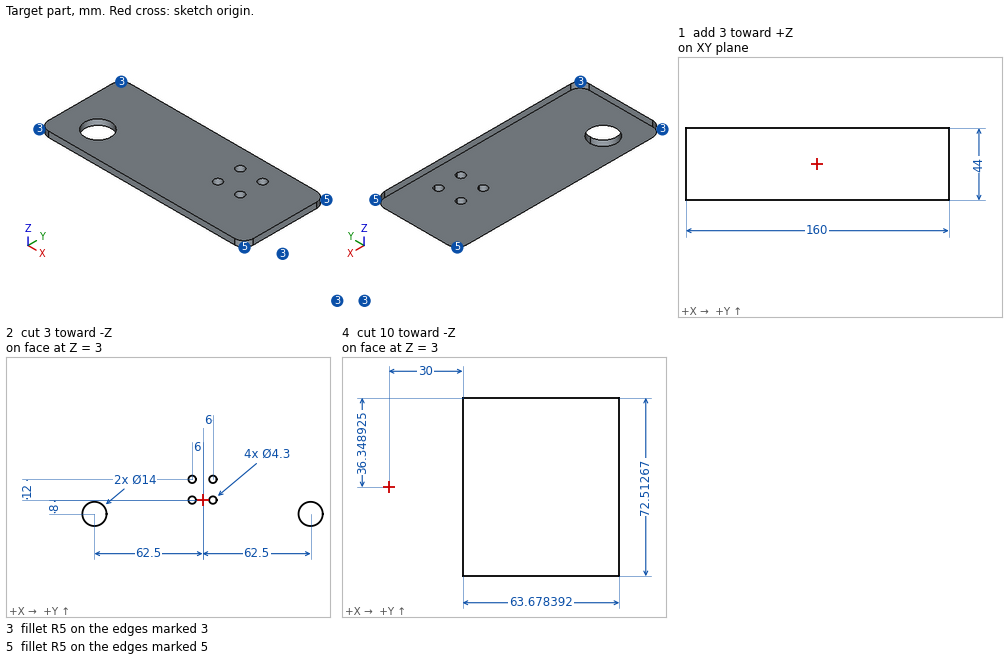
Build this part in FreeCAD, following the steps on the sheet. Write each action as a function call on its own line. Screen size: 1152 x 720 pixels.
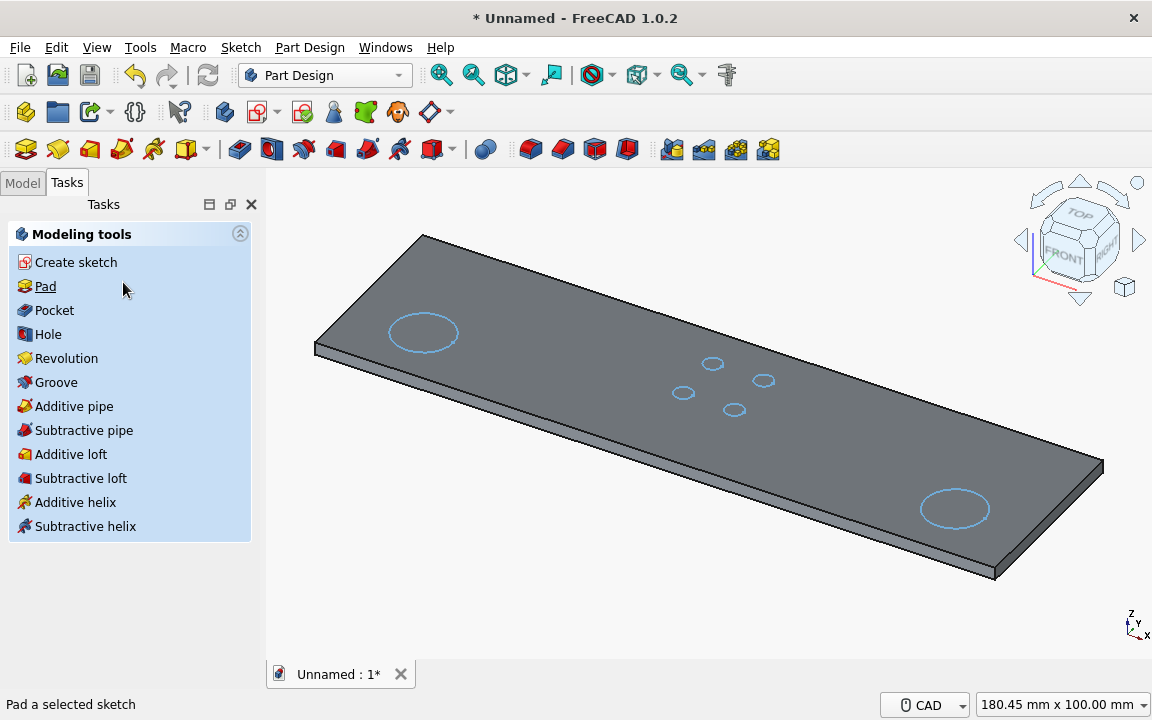
click(240, 150)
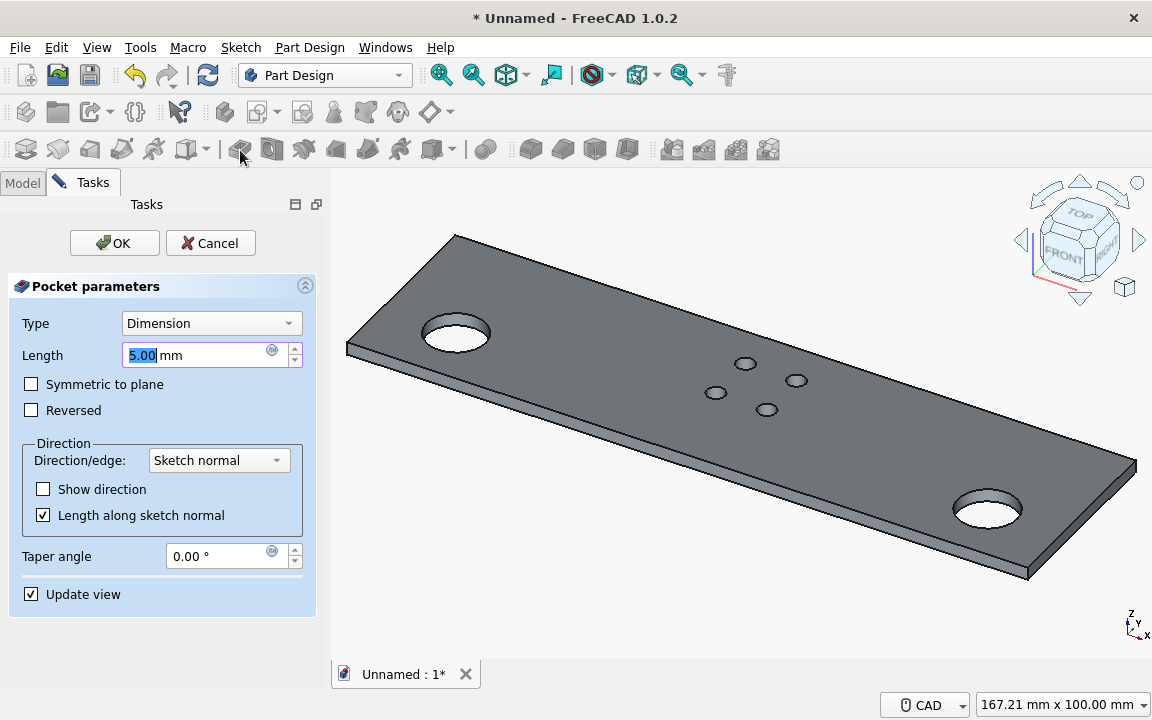
text(3)
key(Tab)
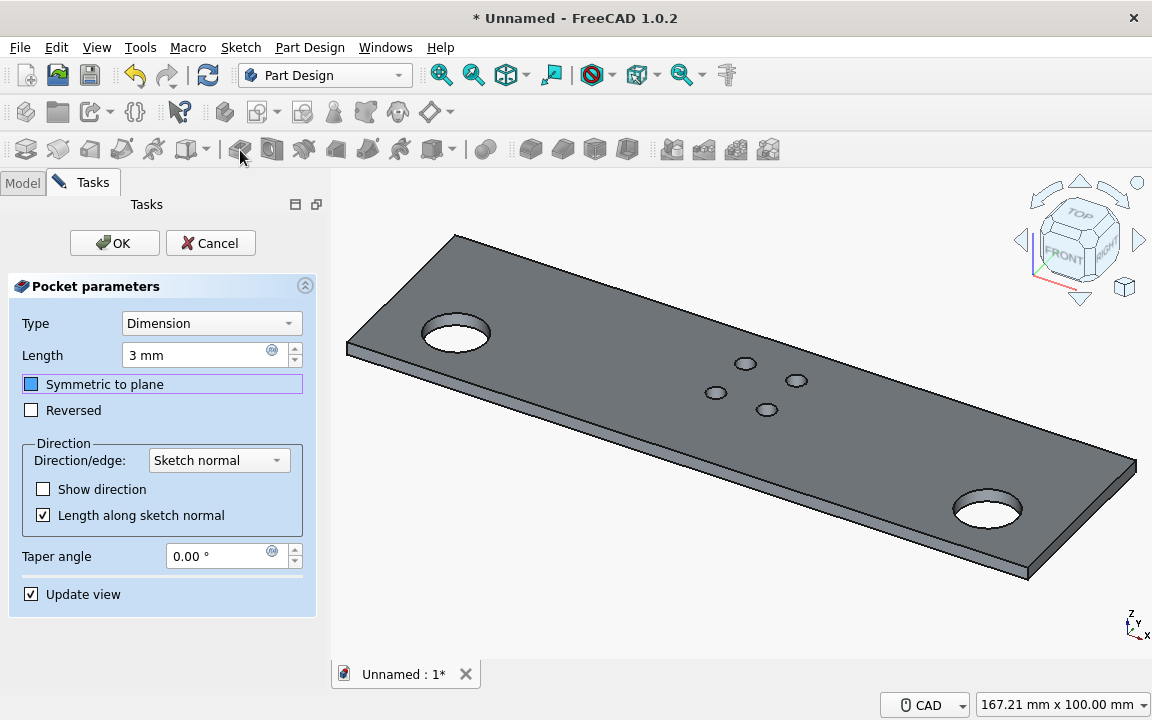
click(115, 243)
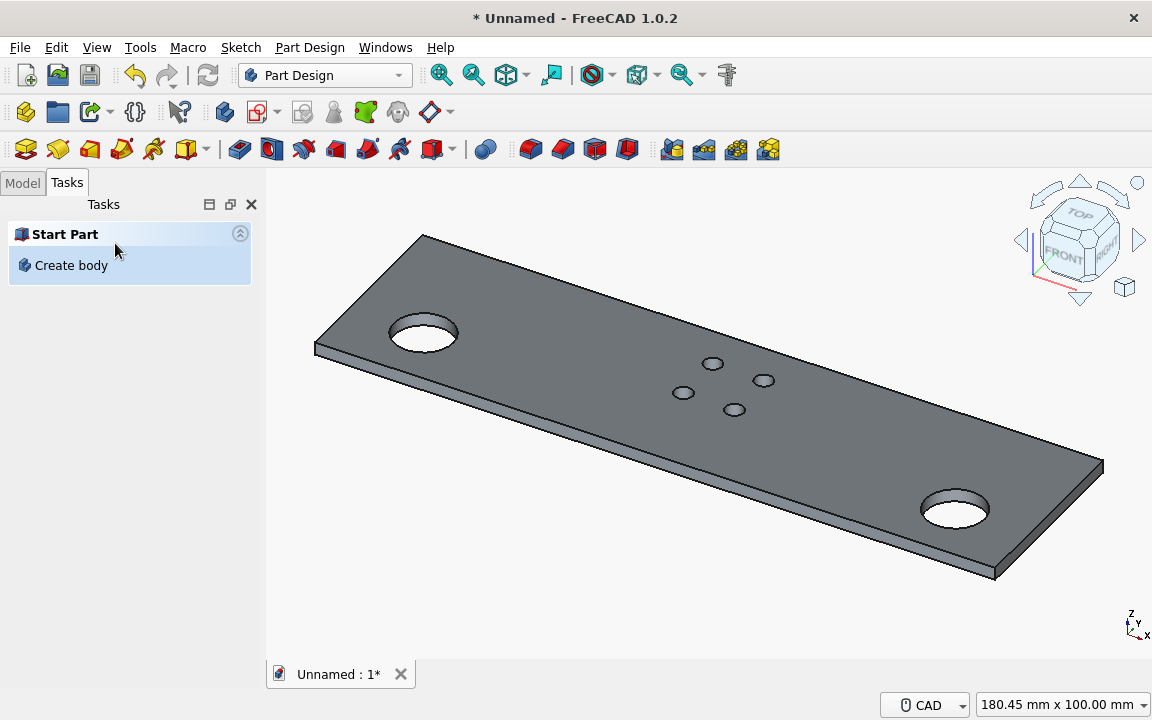
click(995, 573)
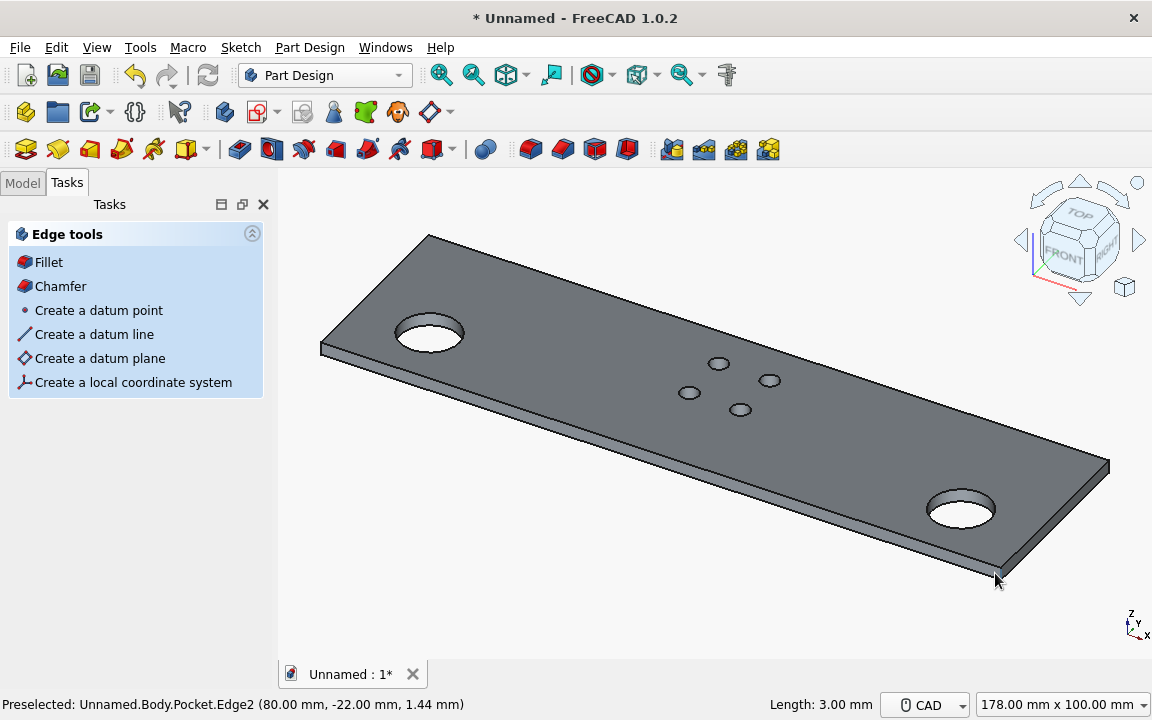
scroll(321, 347, up, 5)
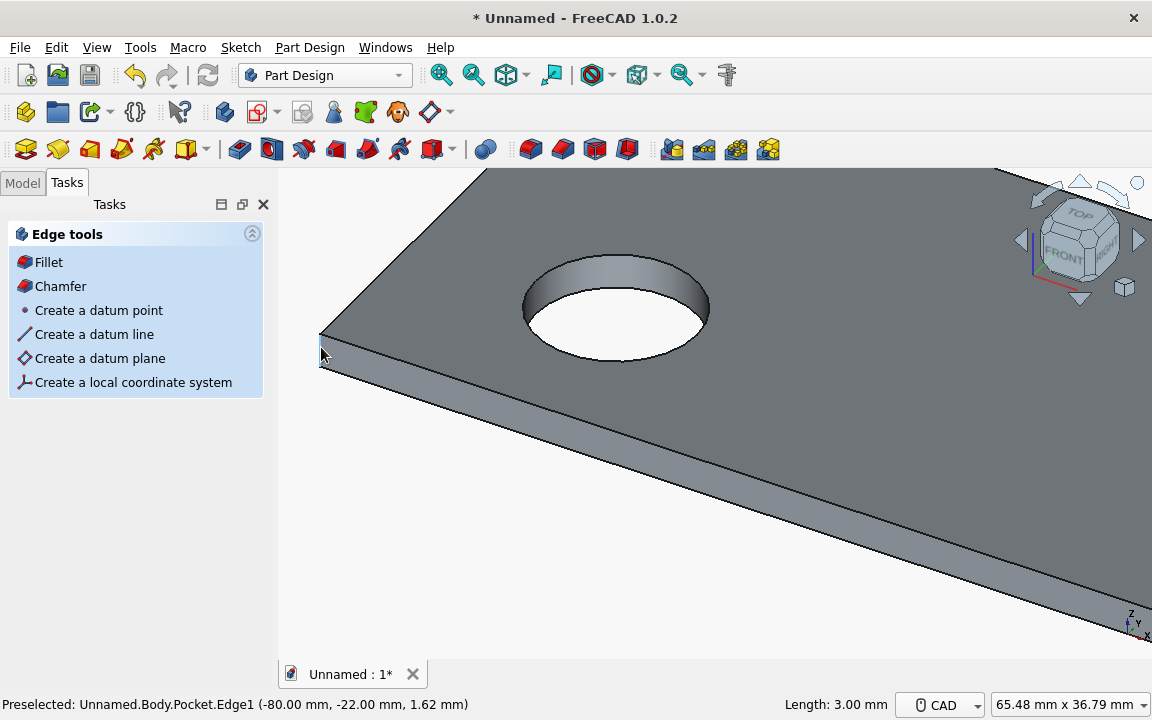
key(v)
key(f)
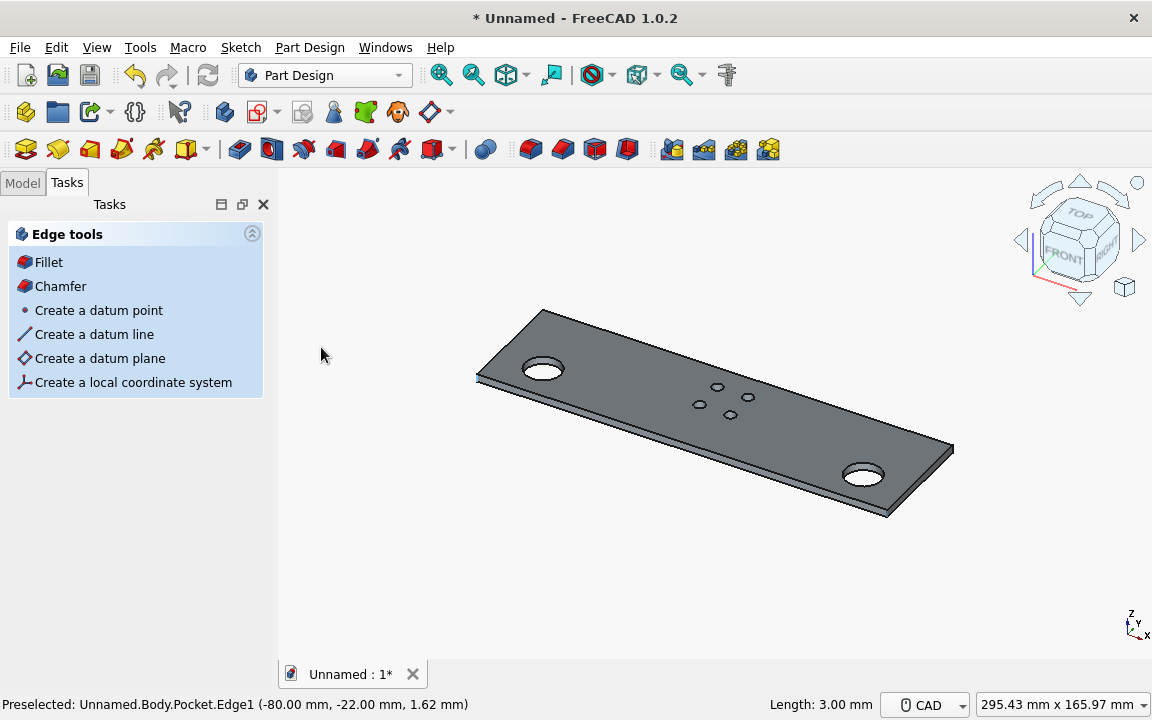
key(0)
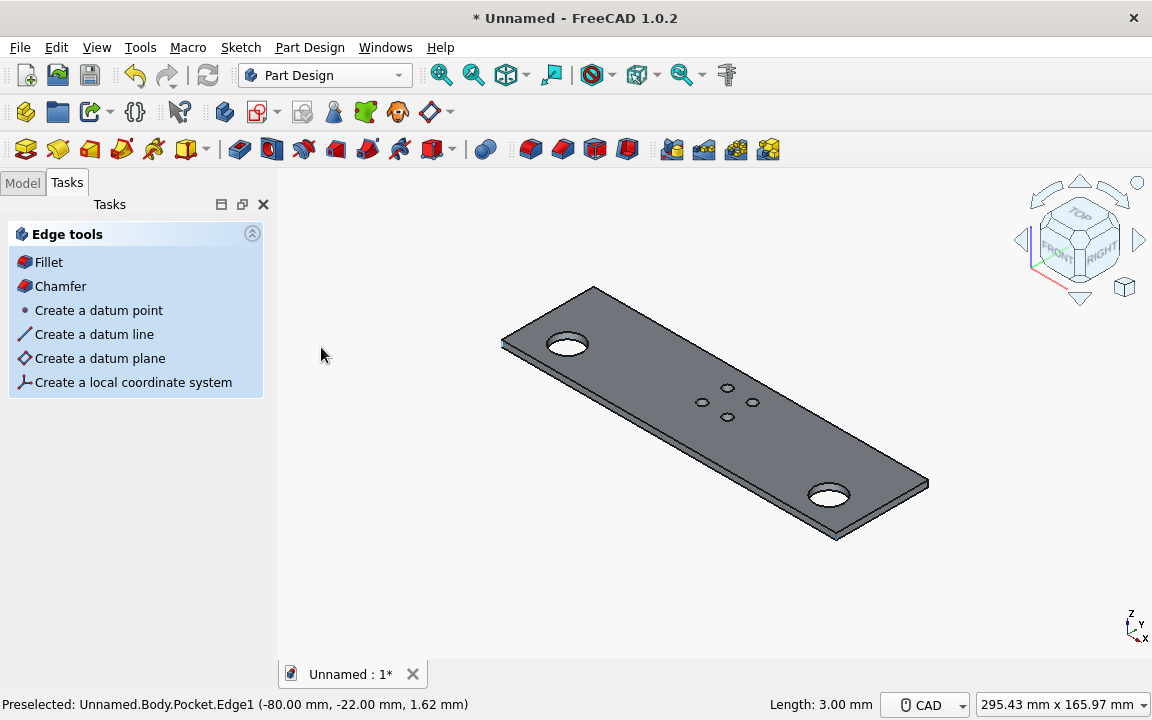
scroll(502, 342, up, 8)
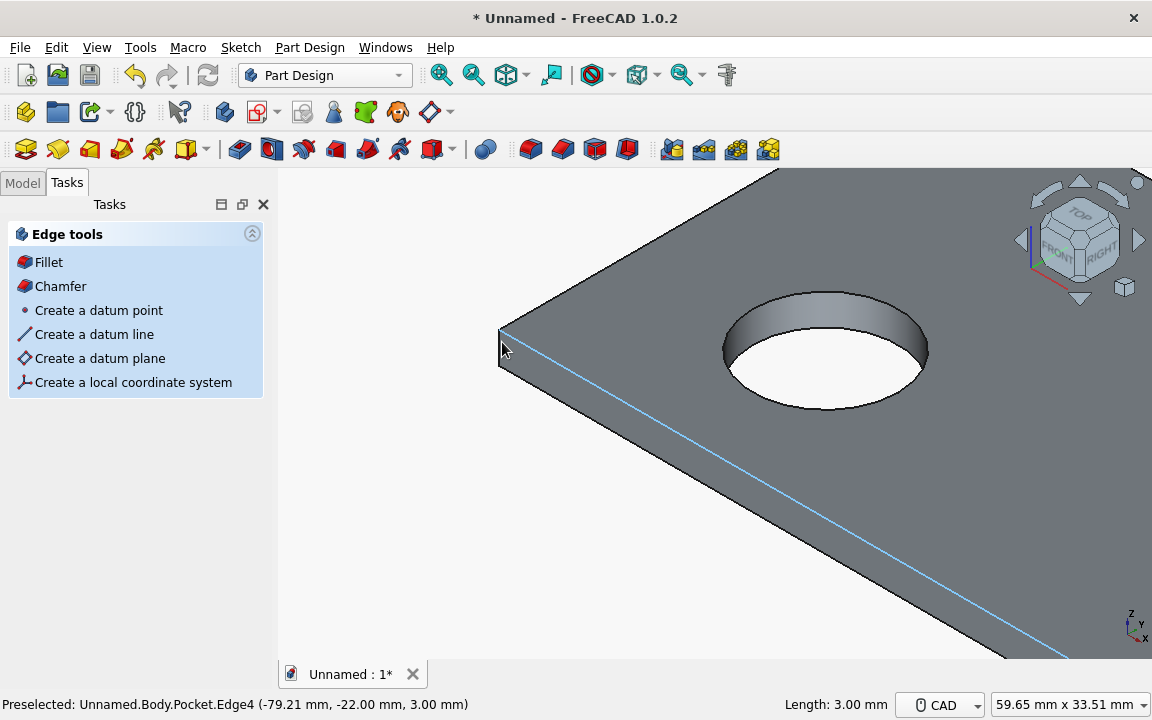
click(442, 76)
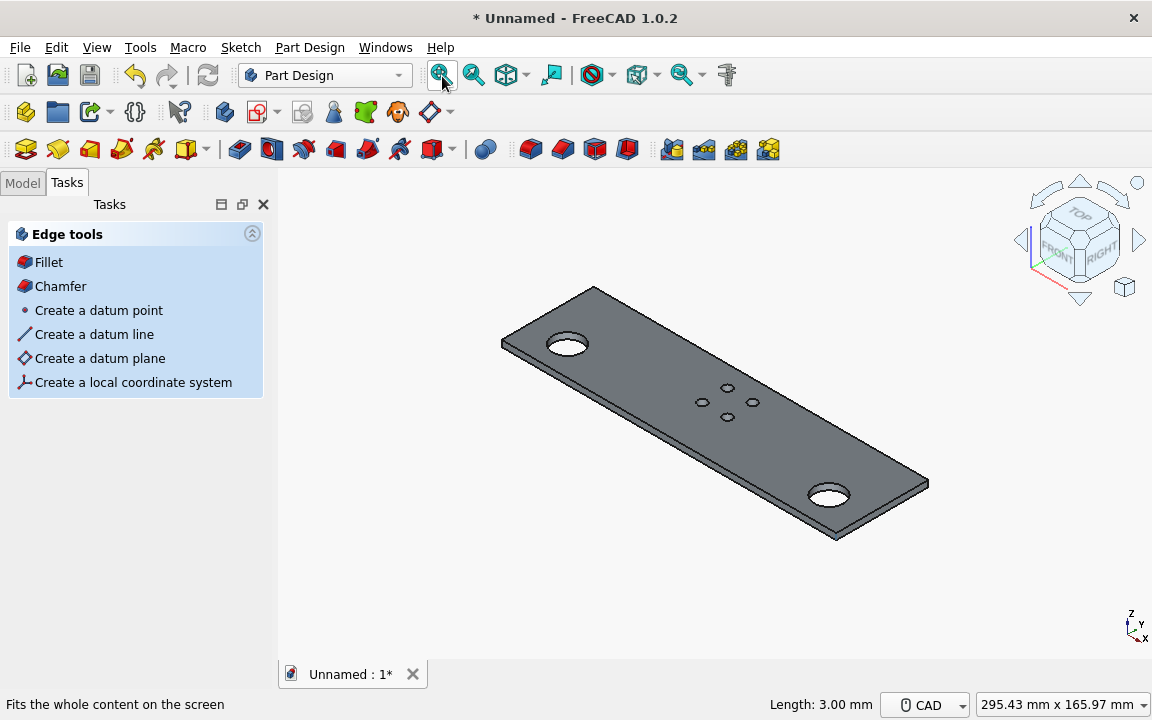
key(2)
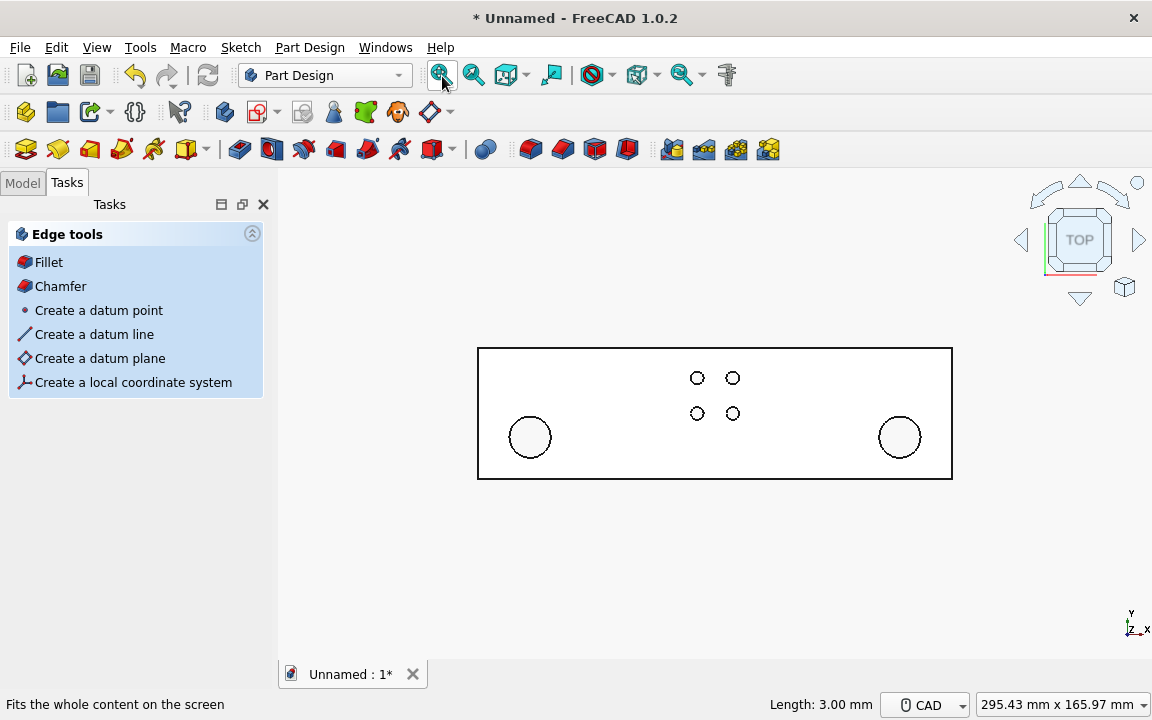
scroll(478, 478, up, 8)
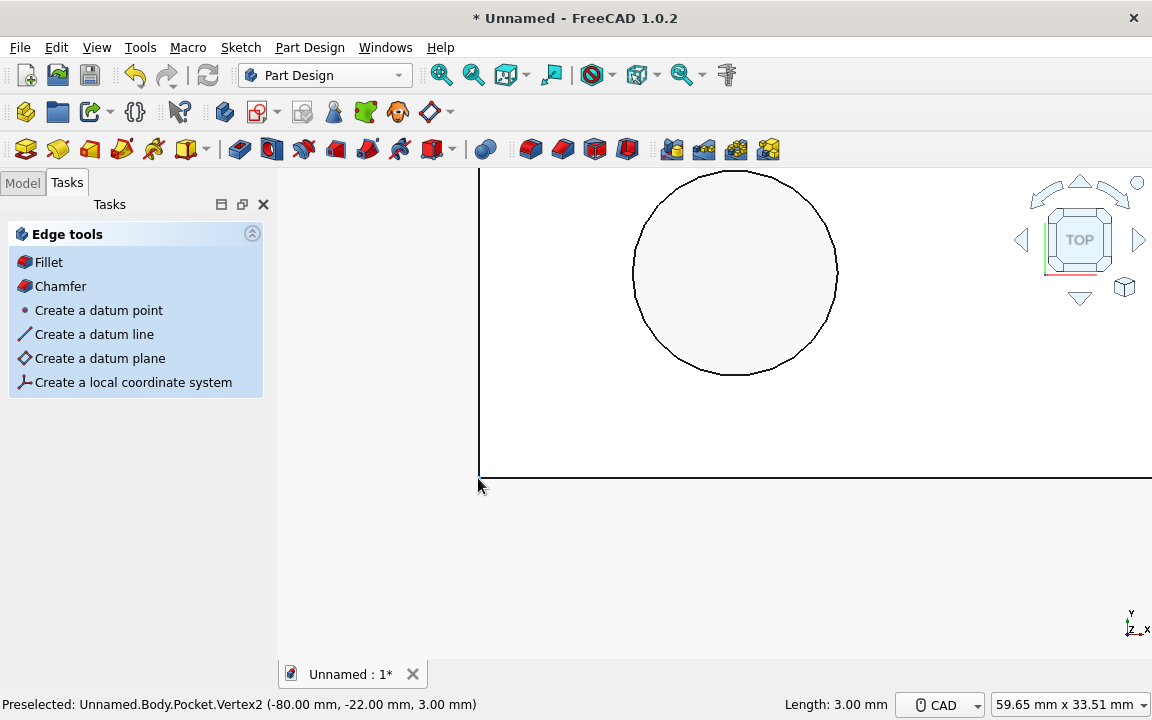
click(442, 76)